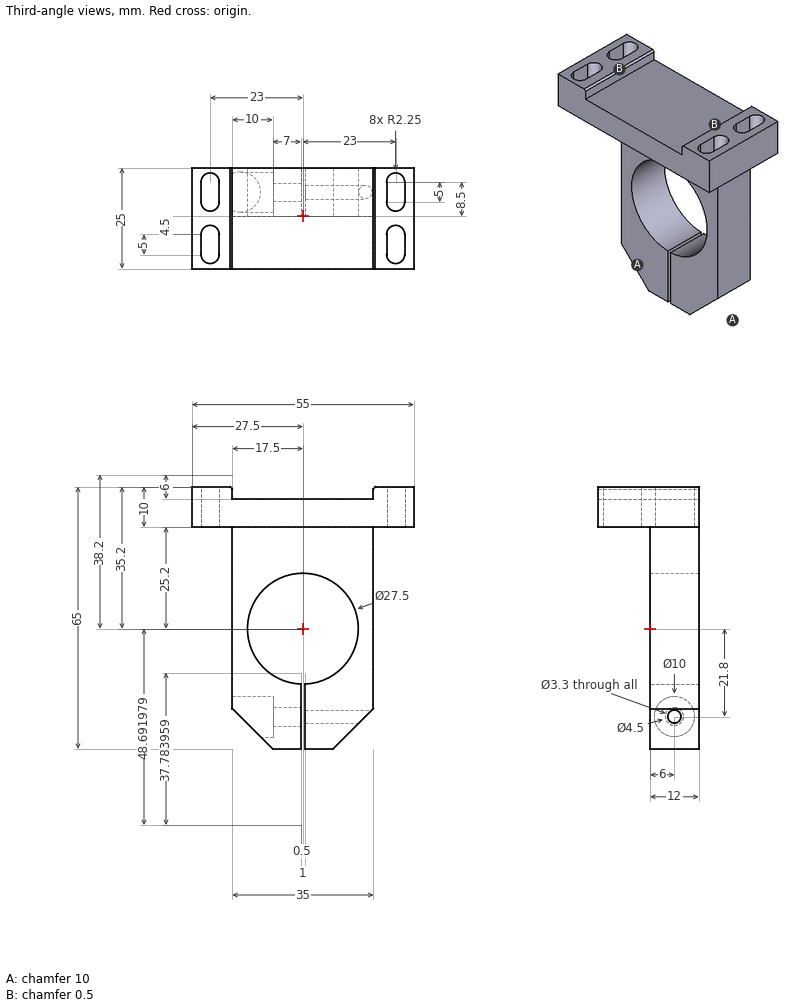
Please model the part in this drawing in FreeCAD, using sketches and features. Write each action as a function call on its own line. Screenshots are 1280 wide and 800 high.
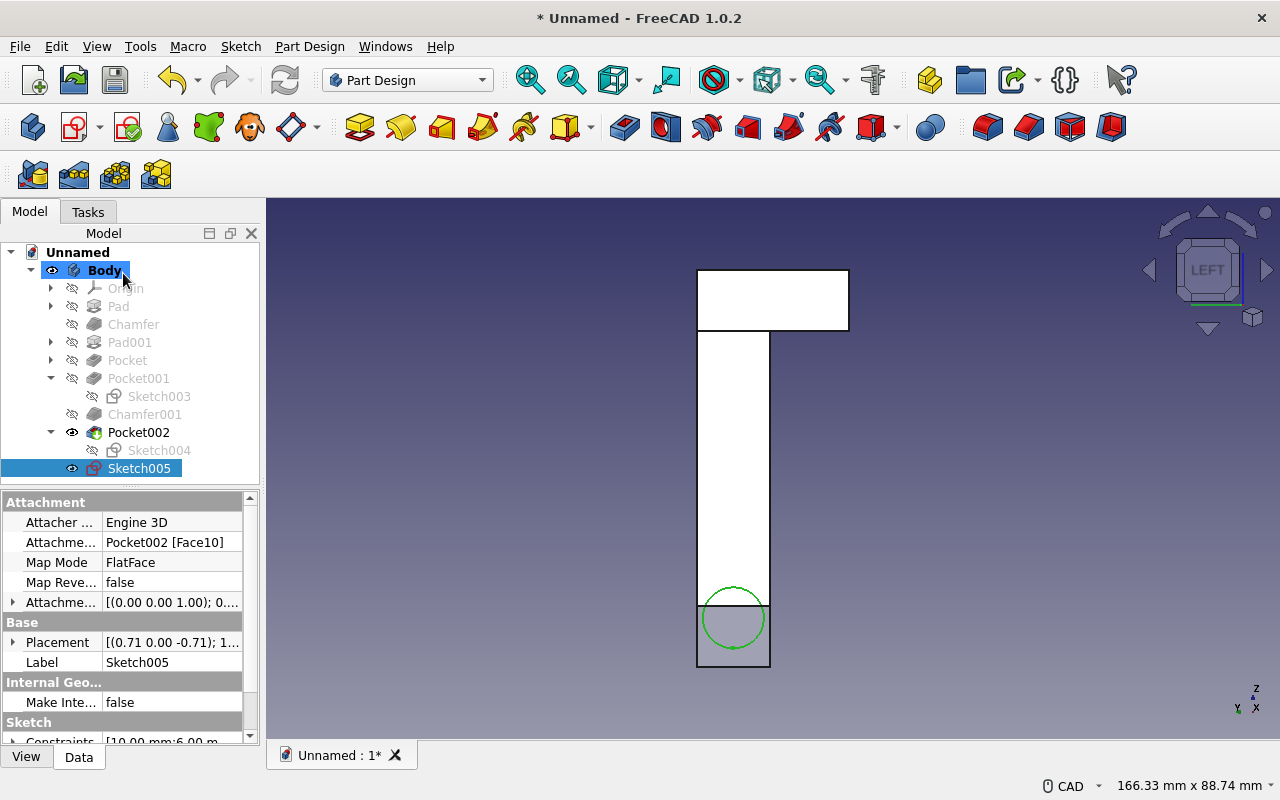
click(625, 128)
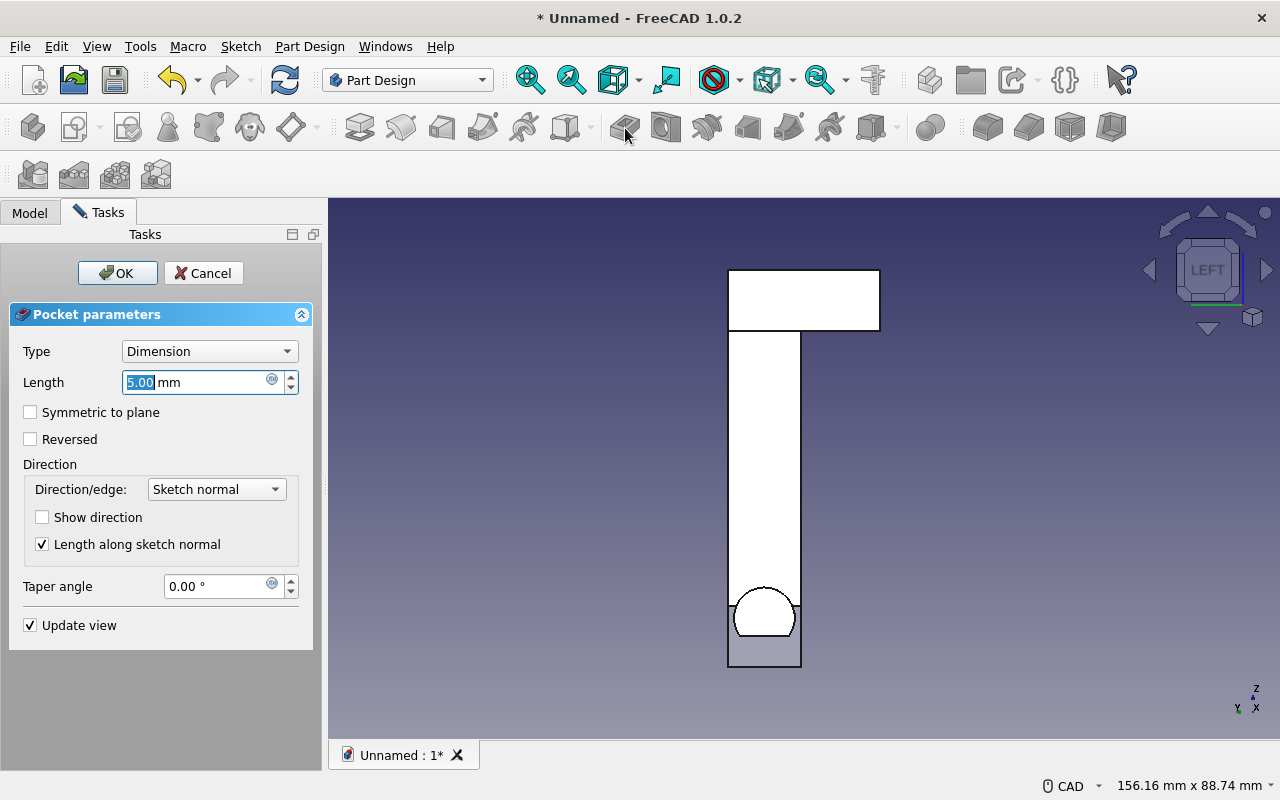
text(10)
key(Tab)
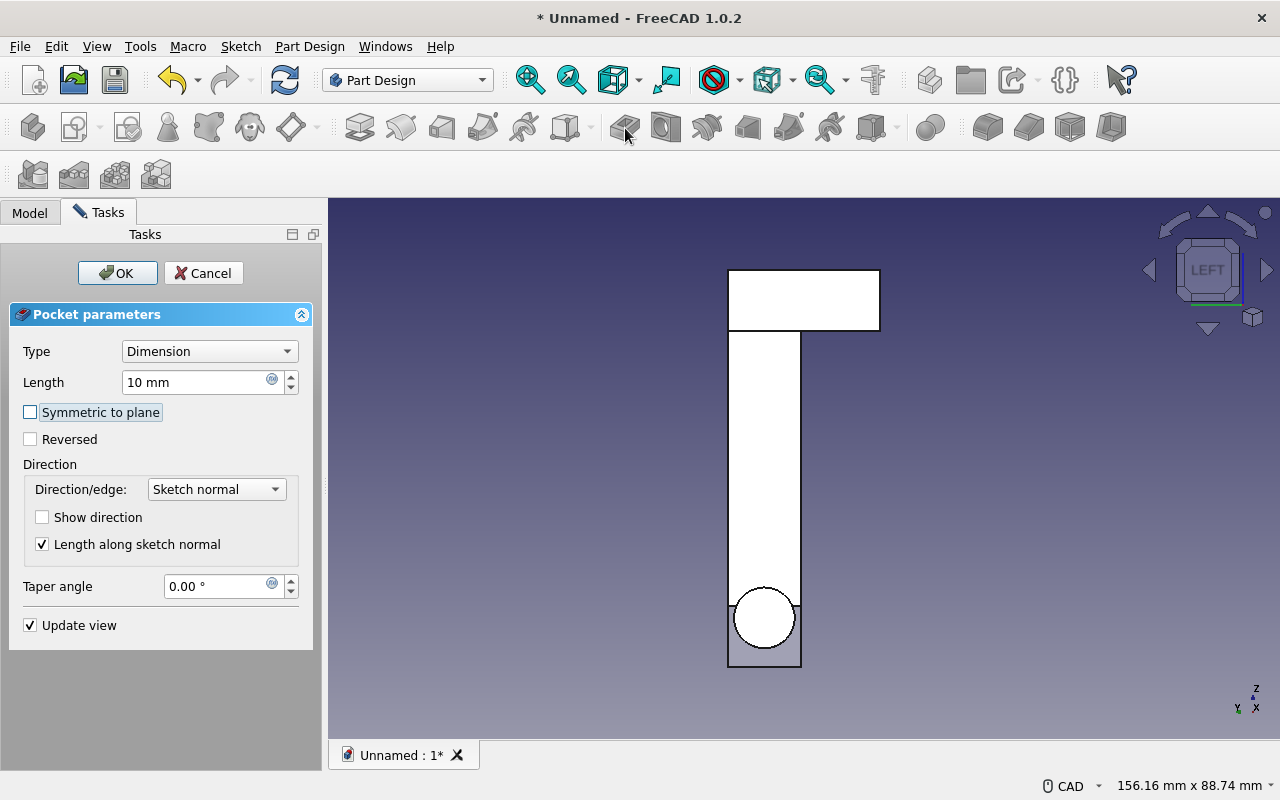
click(118, 273)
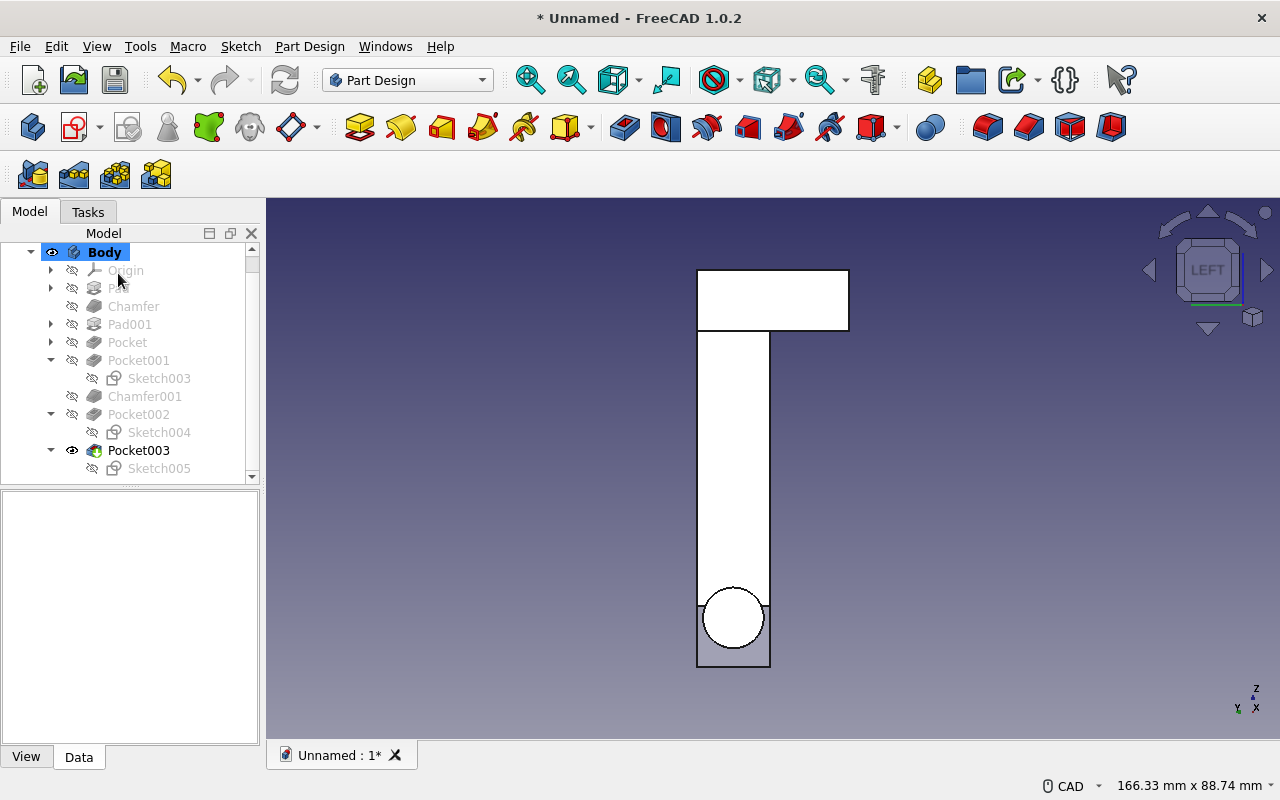
click(733, 617)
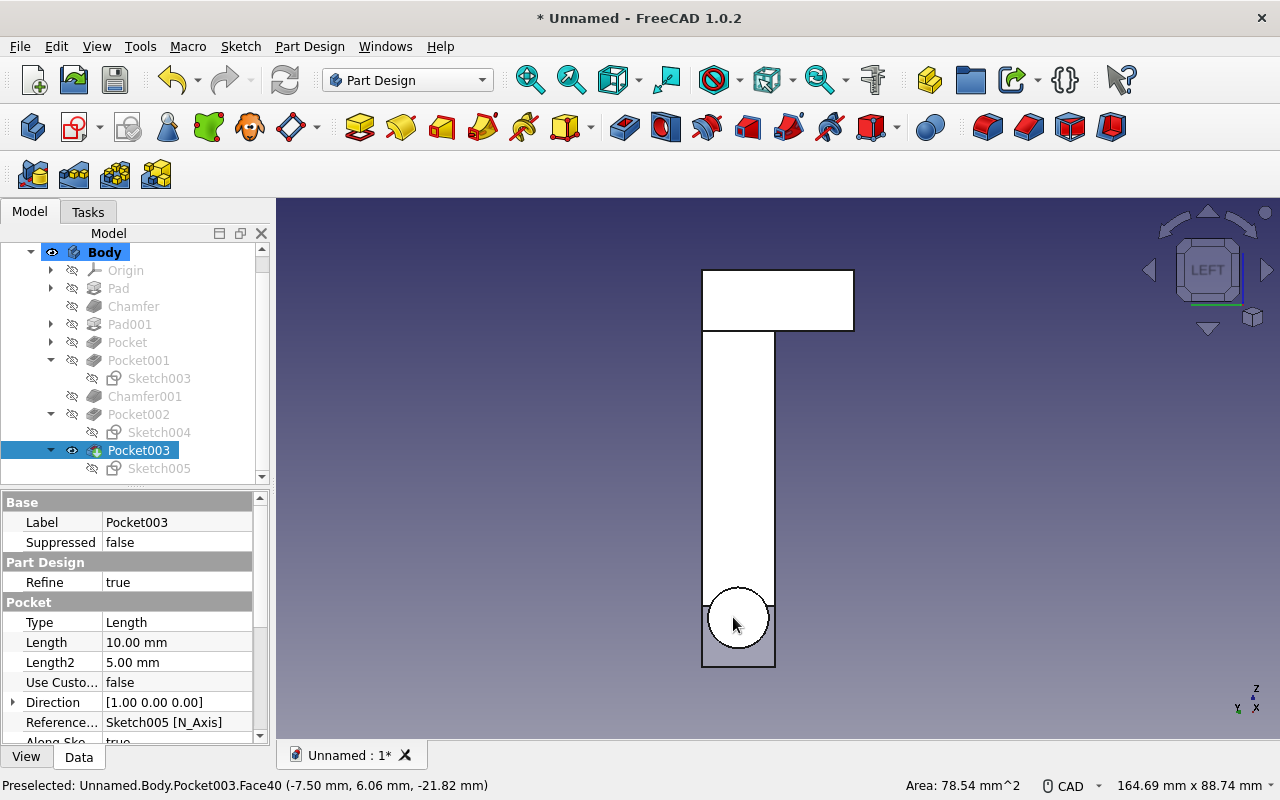
click(74, 128)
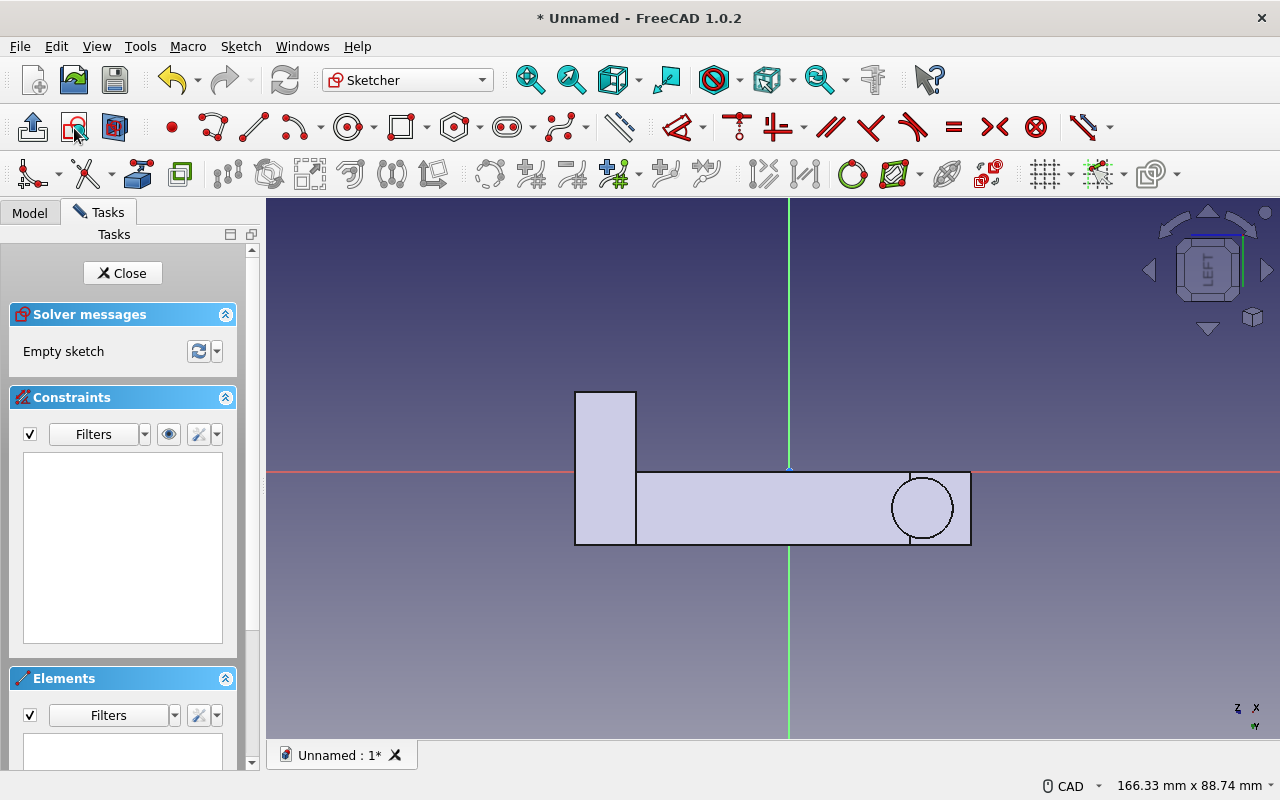
click(115, 128)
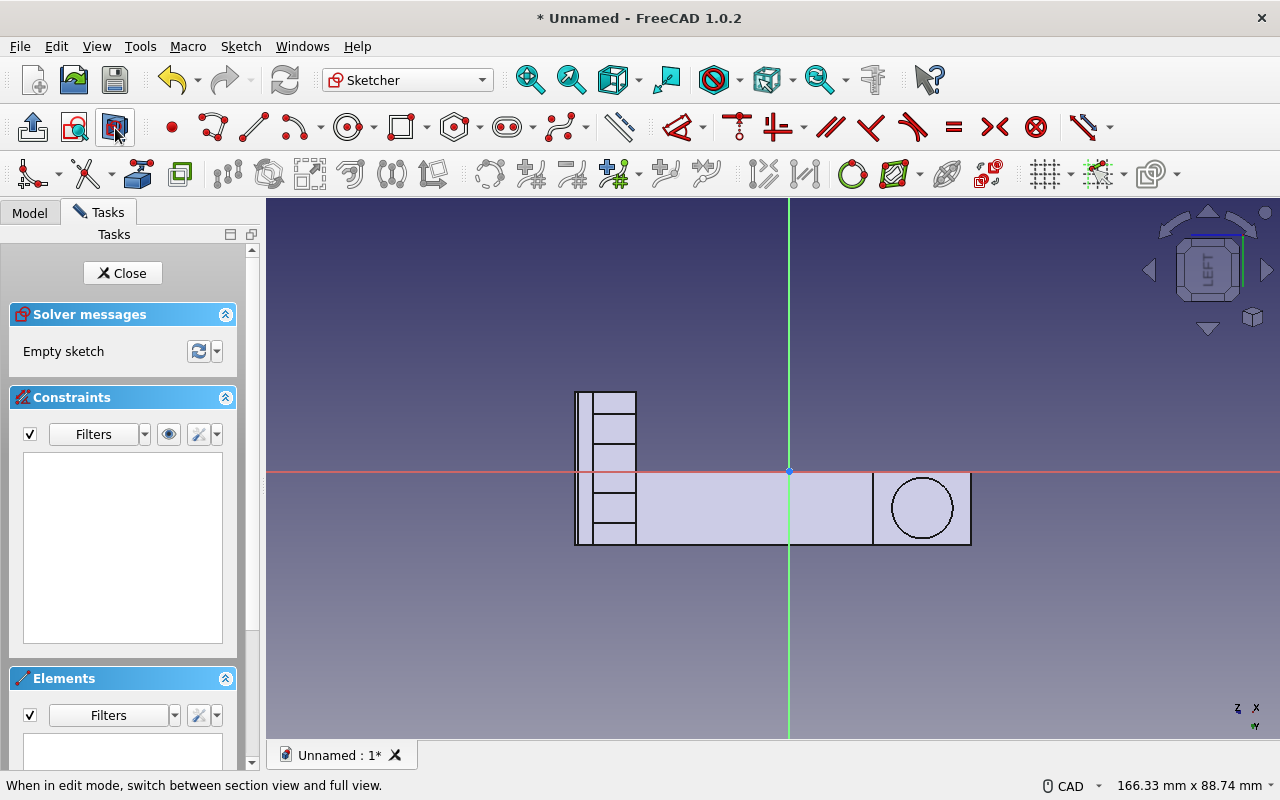
scroll(940, 511, up, 13)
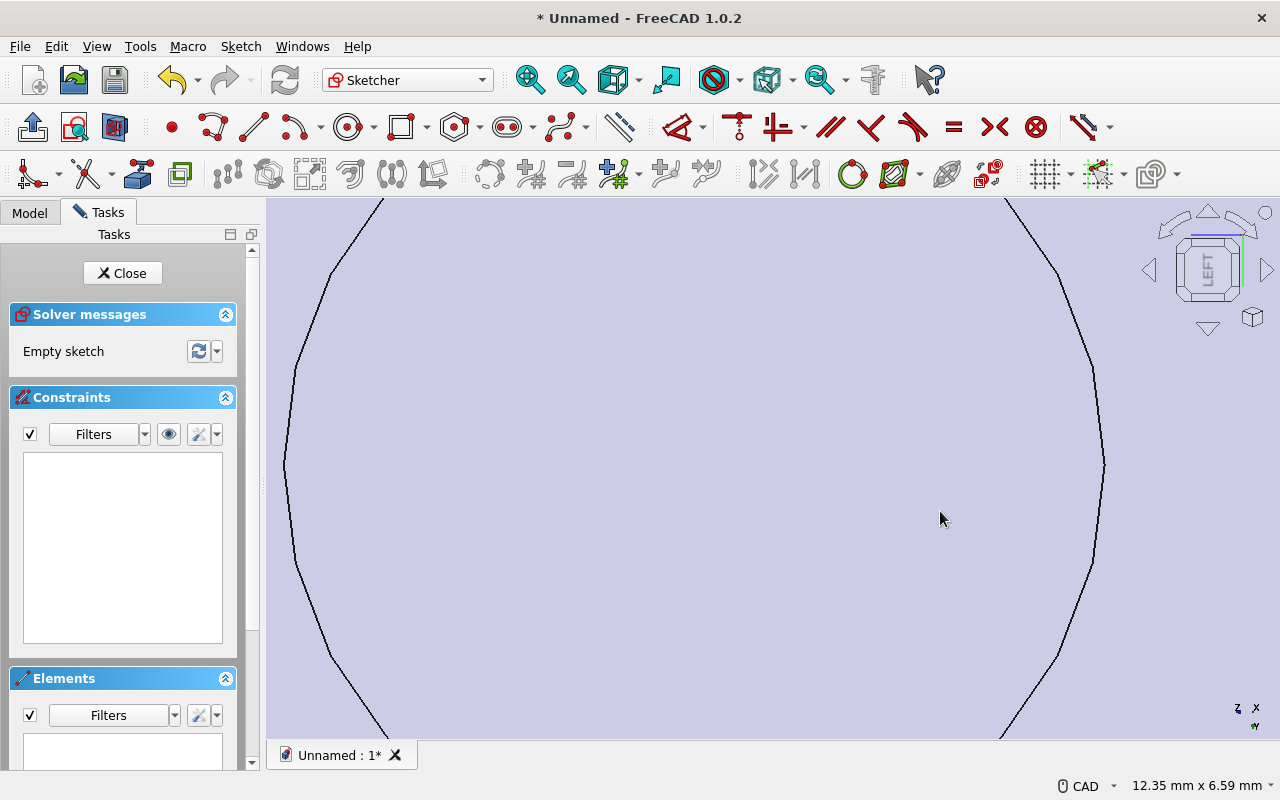
key(g)
key(c)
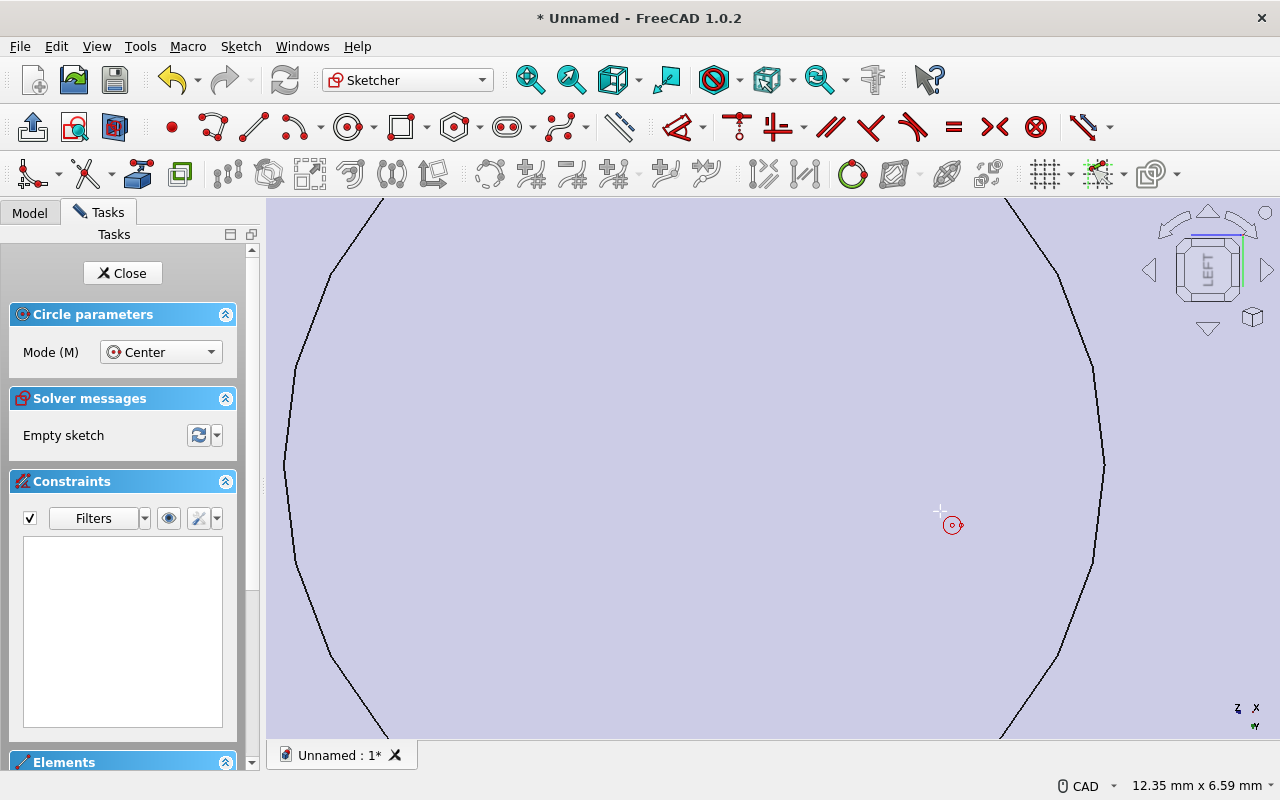
click(694, 465)
click(825, 334)
key(Escape)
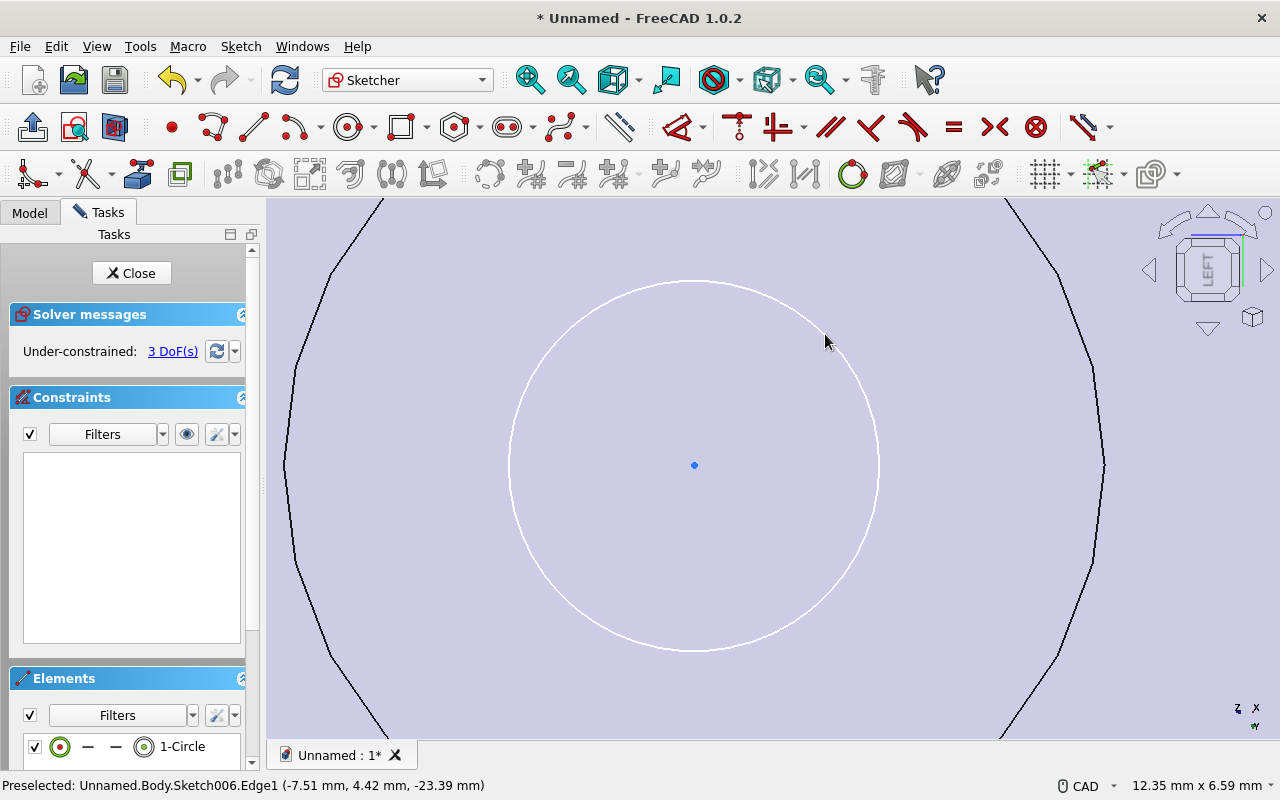
key(d)